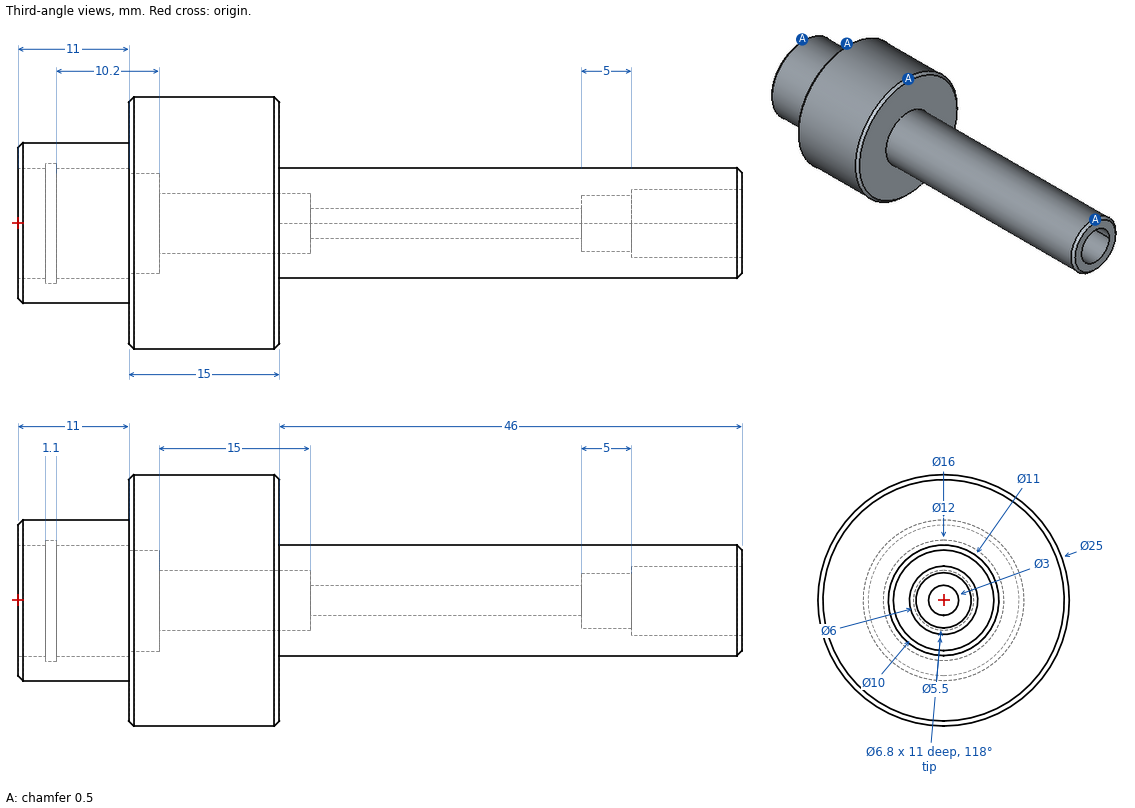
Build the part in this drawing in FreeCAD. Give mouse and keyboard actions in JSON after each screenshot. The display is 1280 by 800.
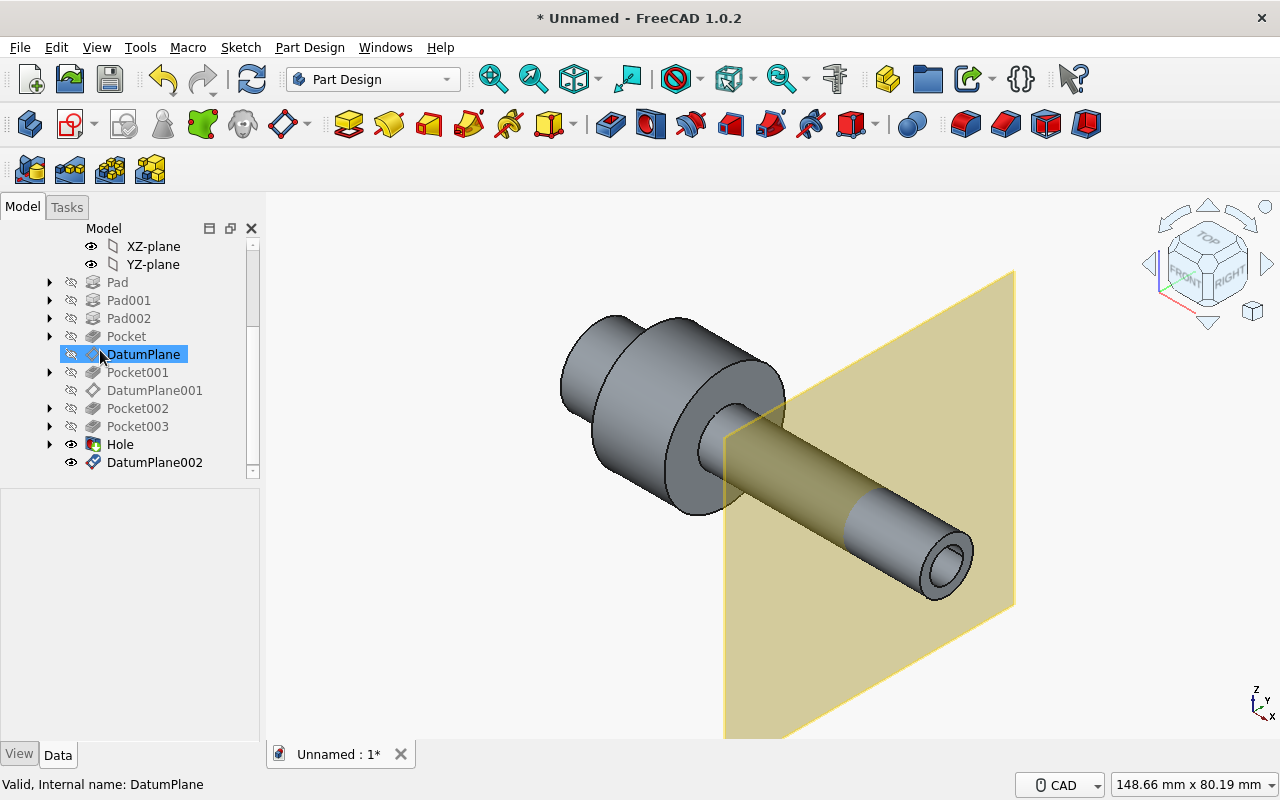
{"action": "left_click", "coordinate": [116, 462]}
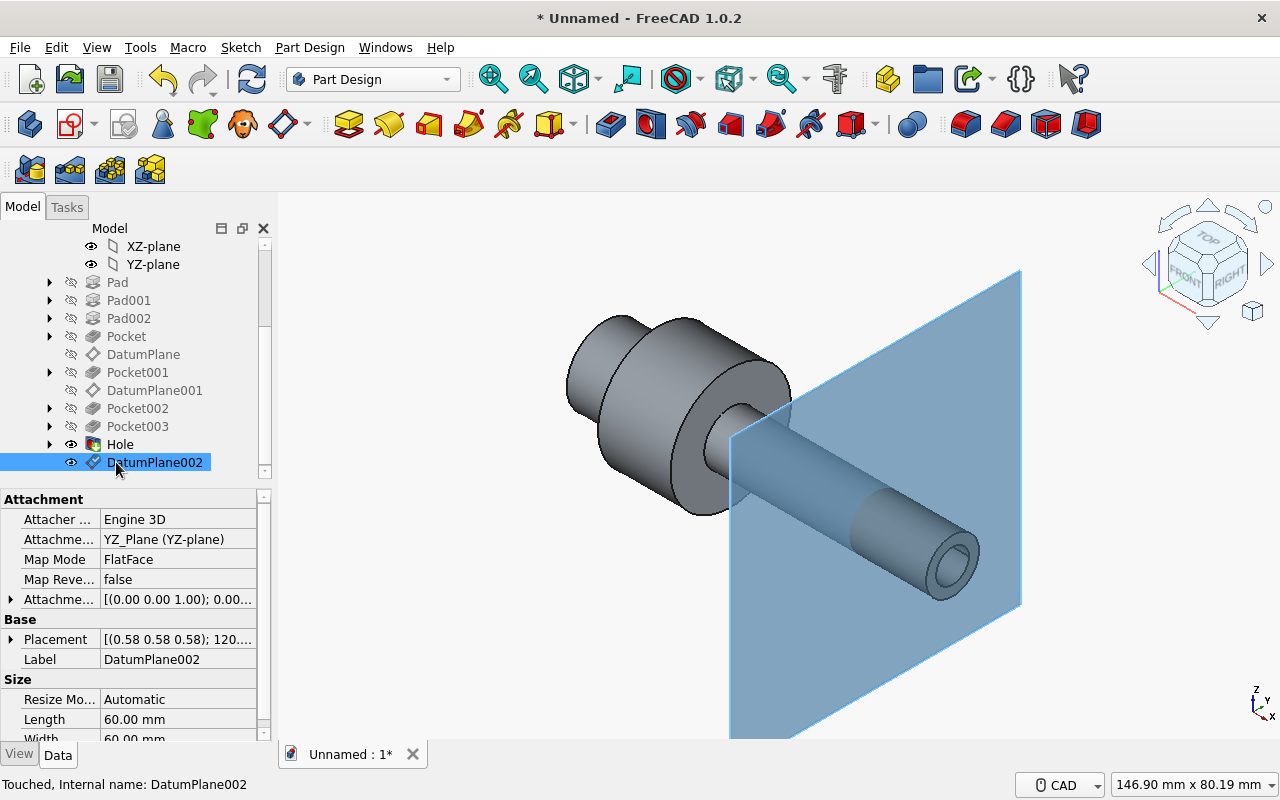
{"action": "left_click", "coordinate": [70, 124]}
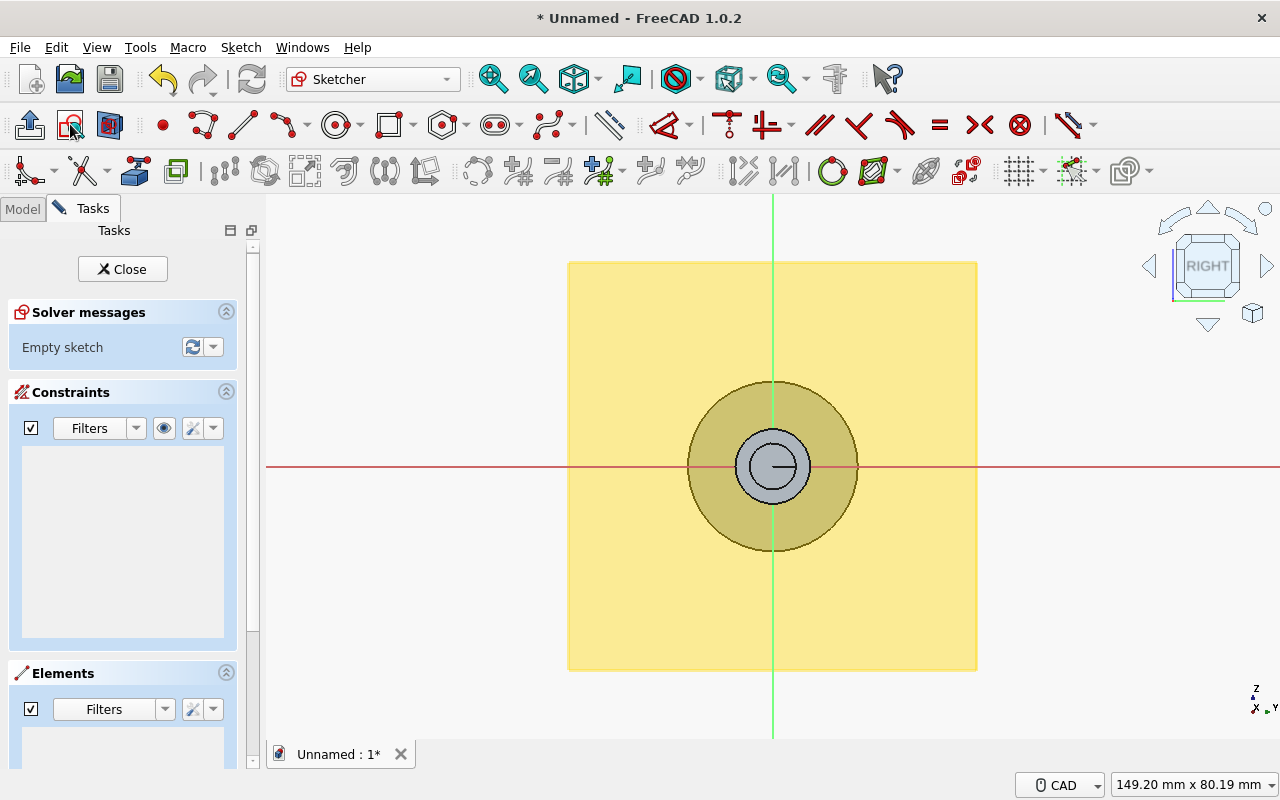
{"action": "key", "text": "q s"}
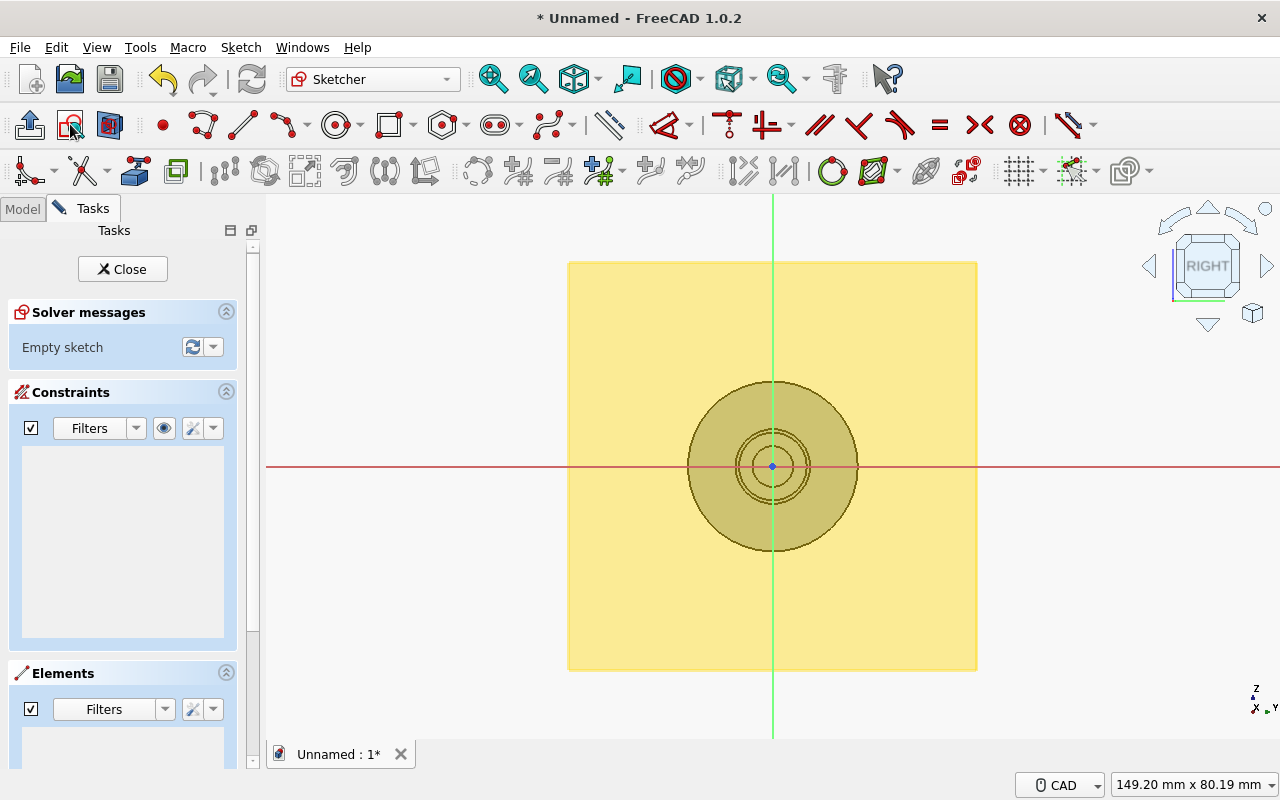
{"action": "scroll", "coordinate": [790, 466], "scroll_direction": "up", "scroll_amount": 8}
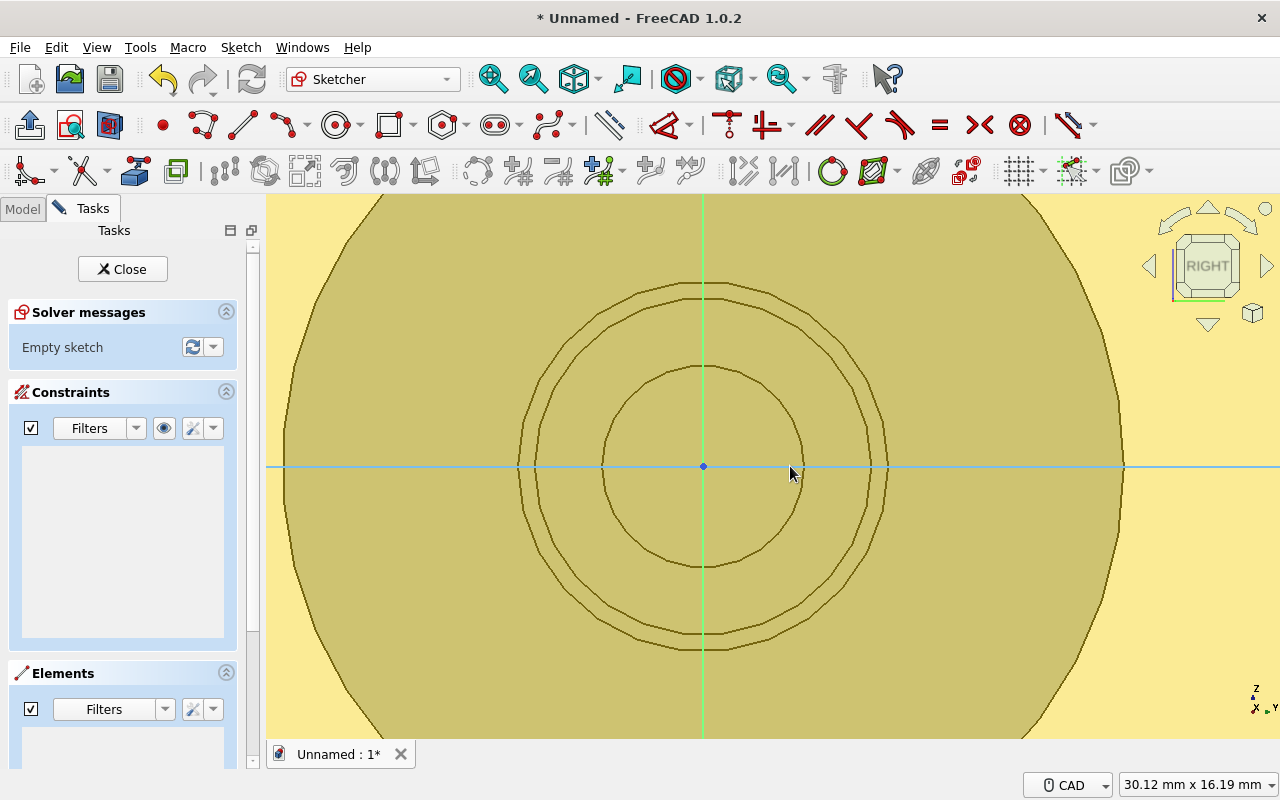
{"action": "left_click", "coordinate": [336, 126]}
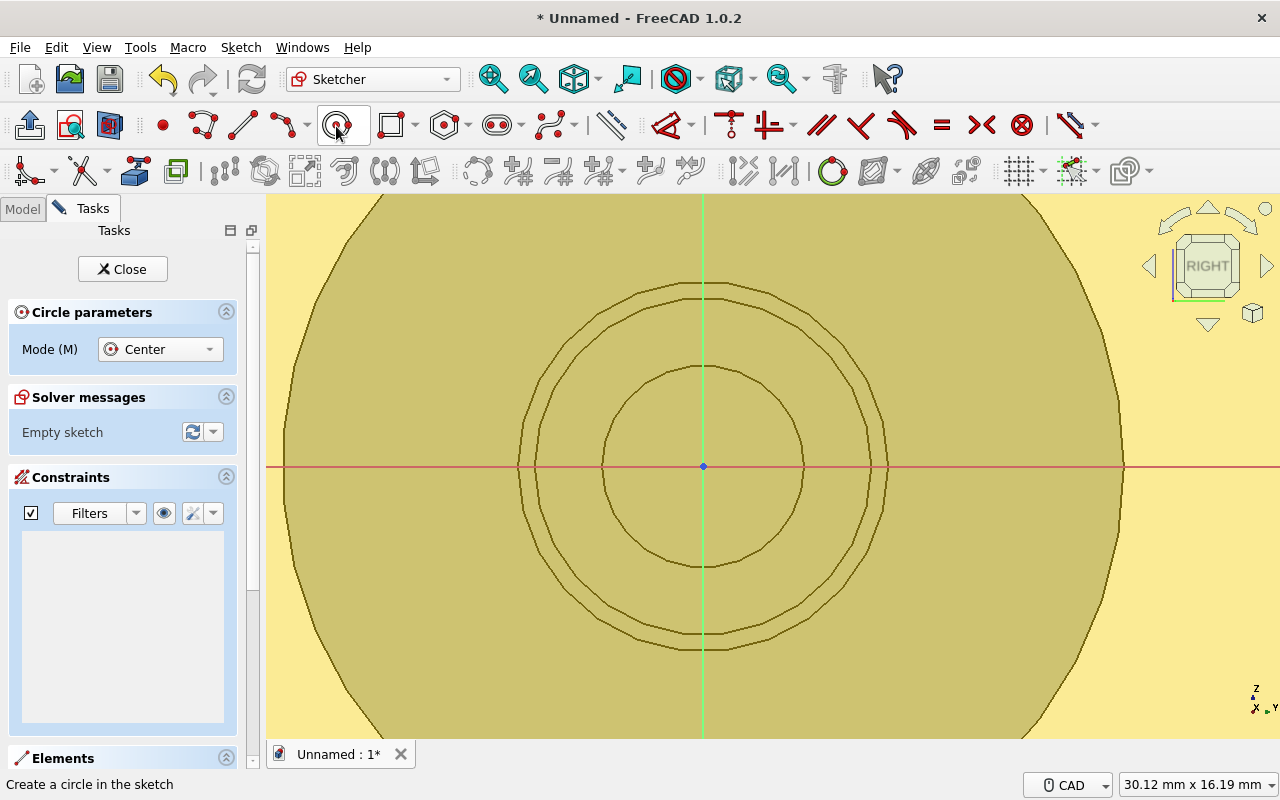
{"action": "left_click", "coordinate": [703, 466]}
{"action": "mouse_move", "coordinate": [834, 336]}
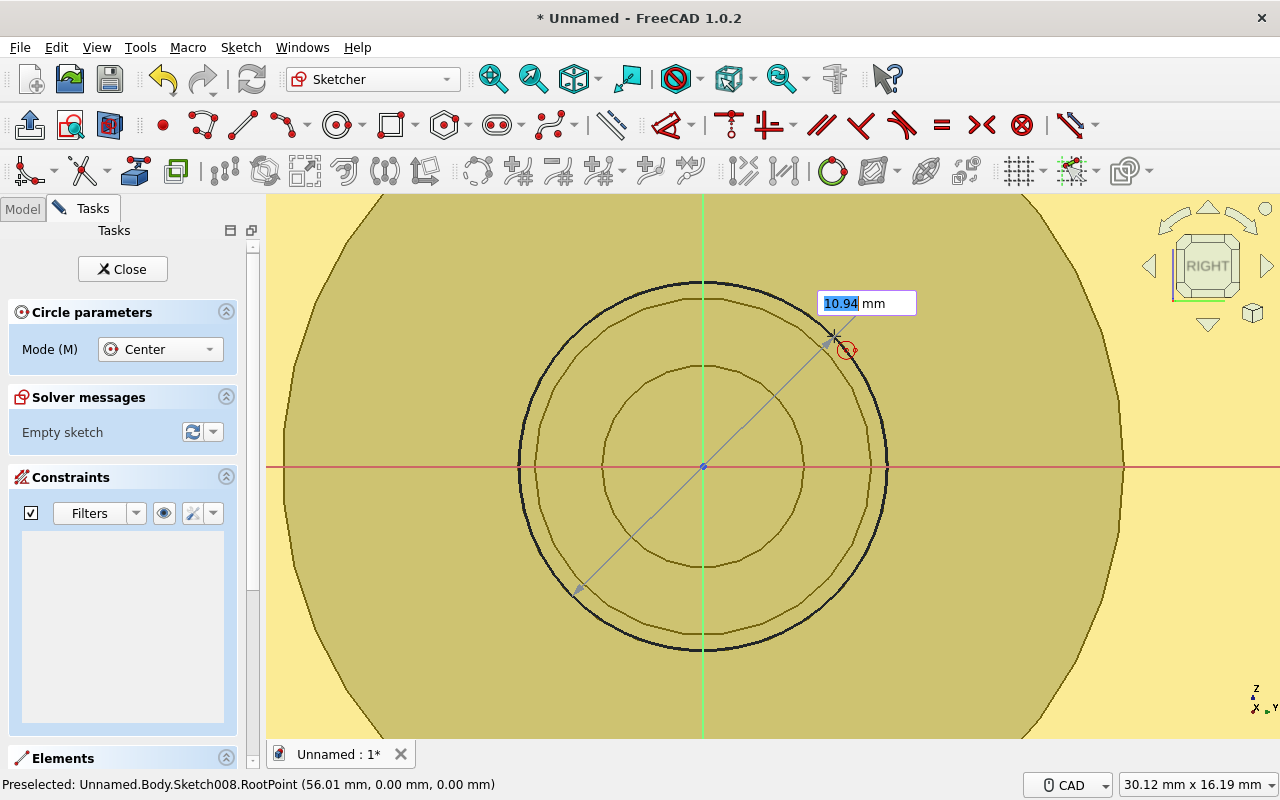
{"action": "type", "text": "11"}
{"action": "key", "text": "Return"}
{"action": "key", "text": "Escape"}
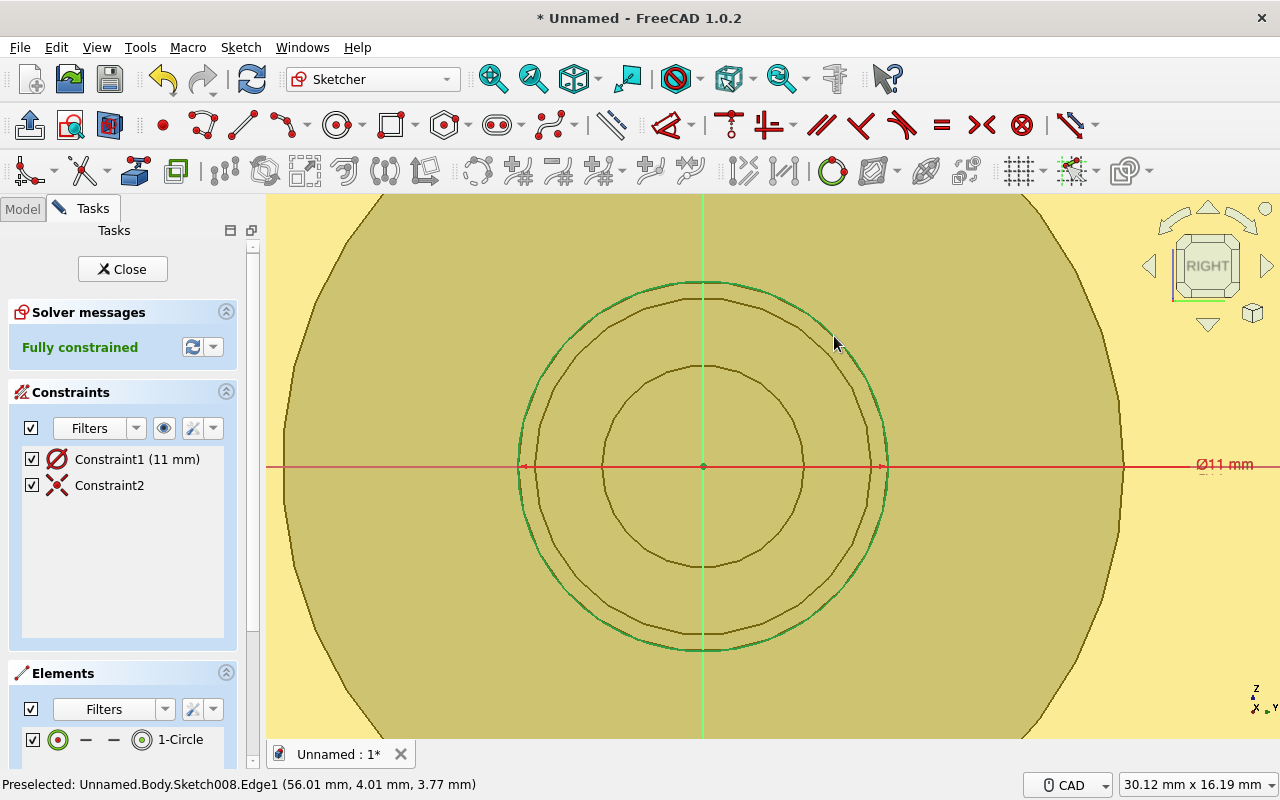
{"action": "left_click", "coordinate": [123, 269]}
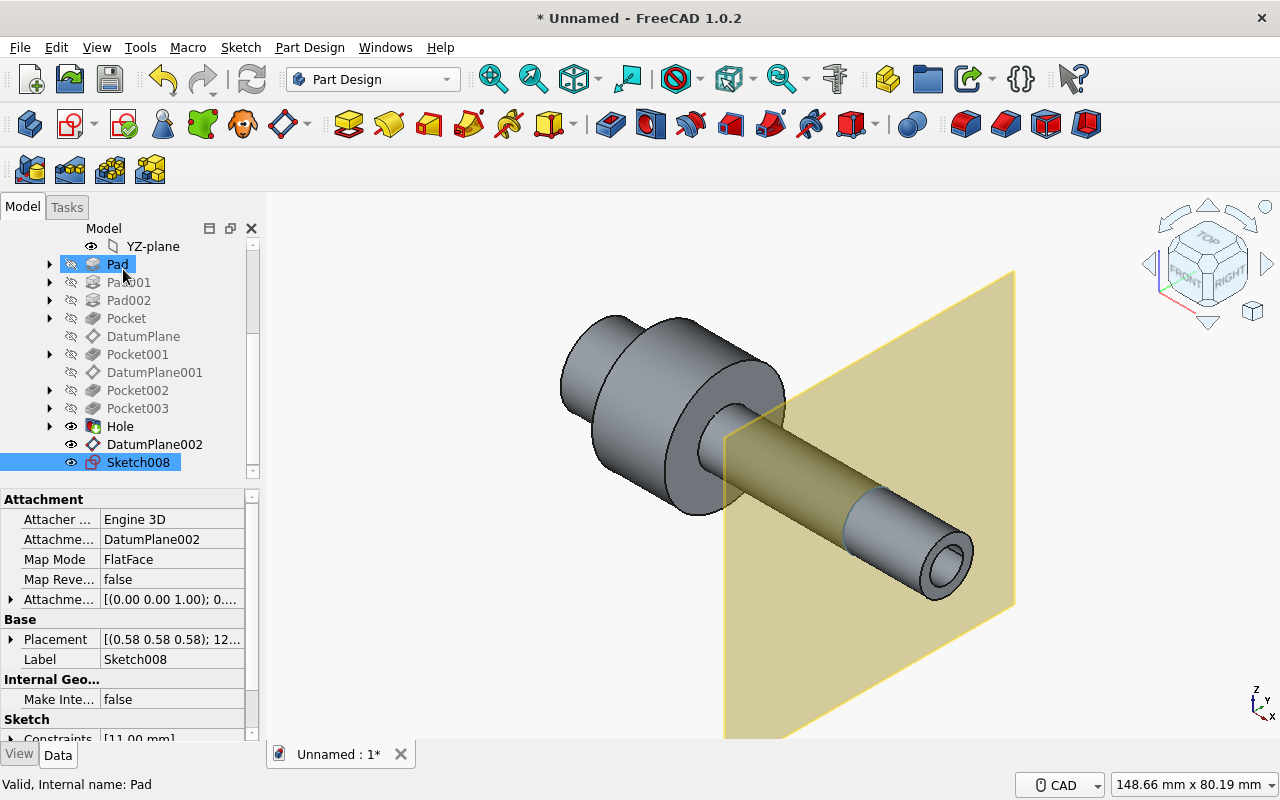
{"action": "left_click", "coordinate": [350, 124]}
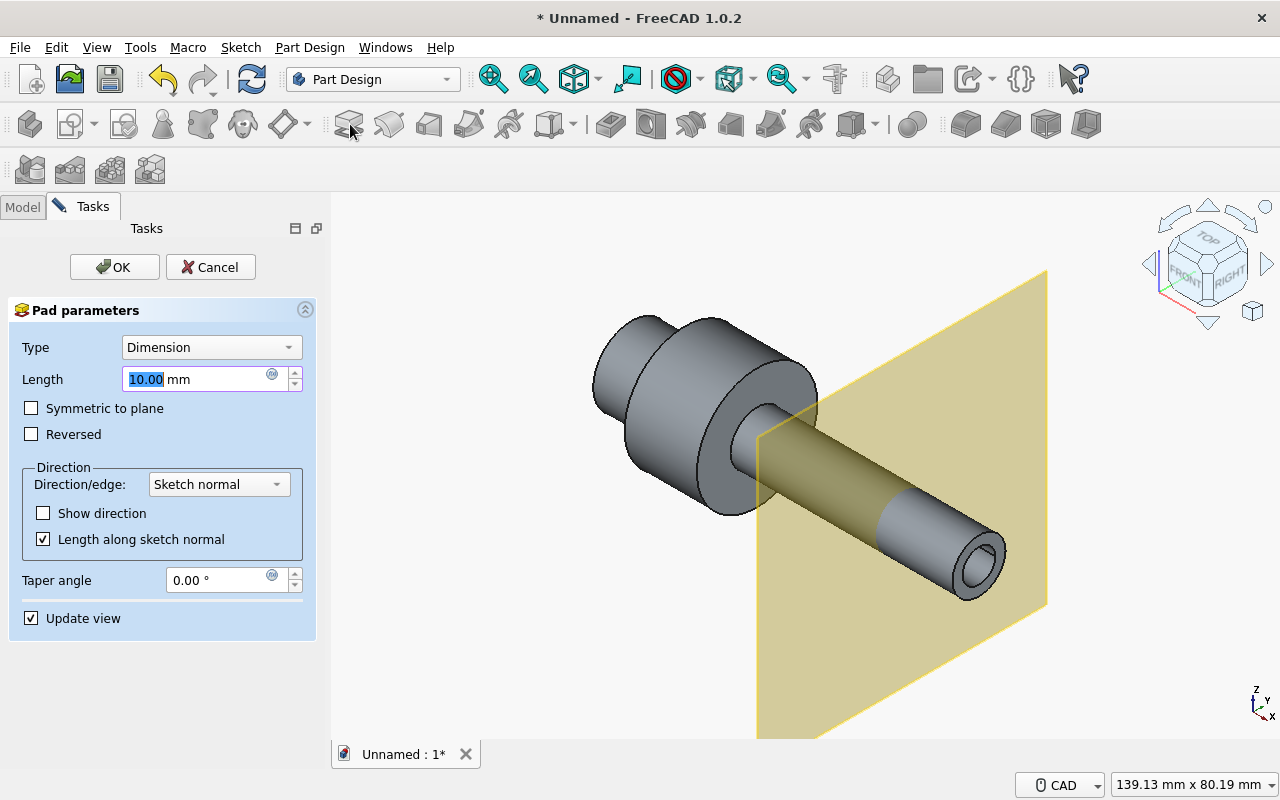
{"action": "type", "text": "5"}
{"action": "key", "text": "Tab"}